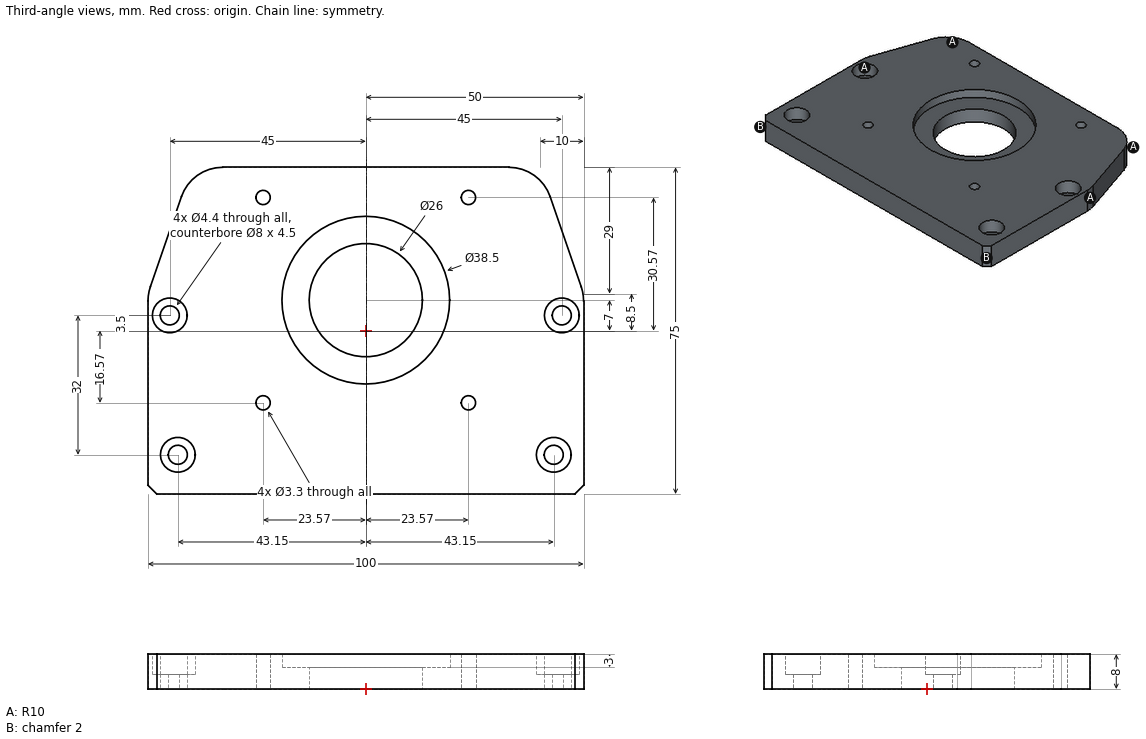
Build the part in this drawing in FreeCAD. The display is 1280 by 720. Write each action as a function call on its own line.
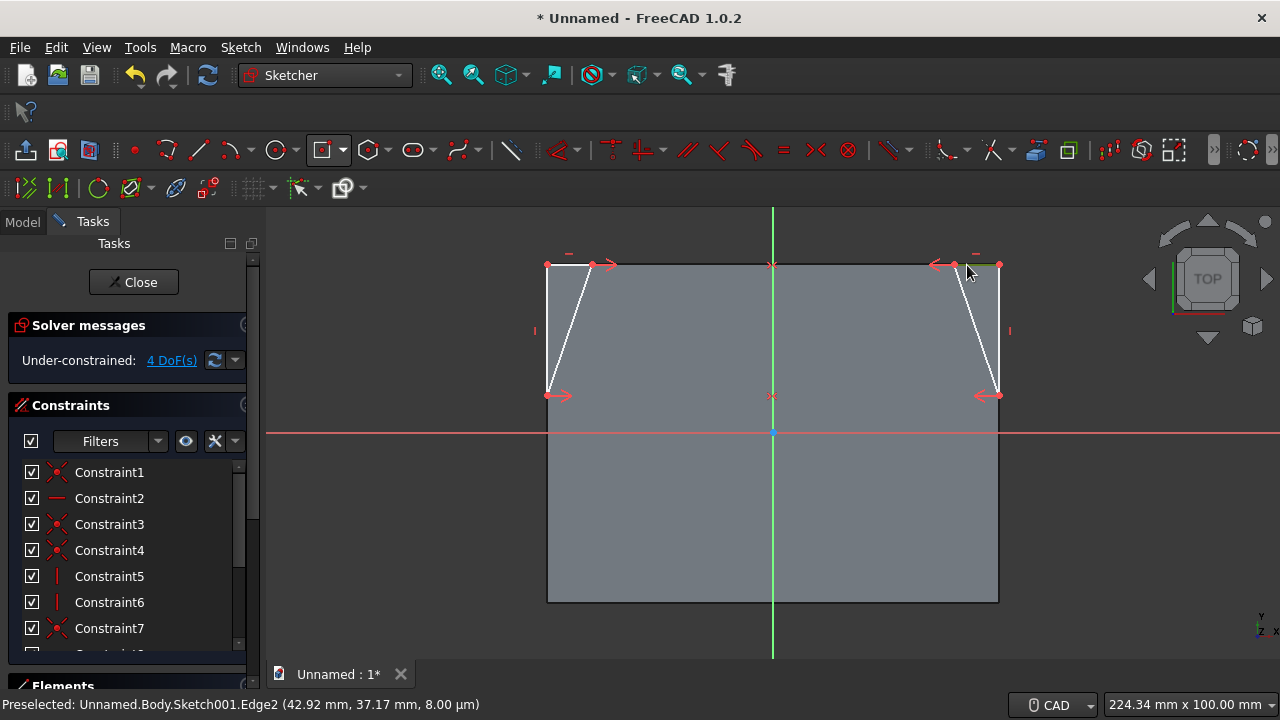
click(580, 150)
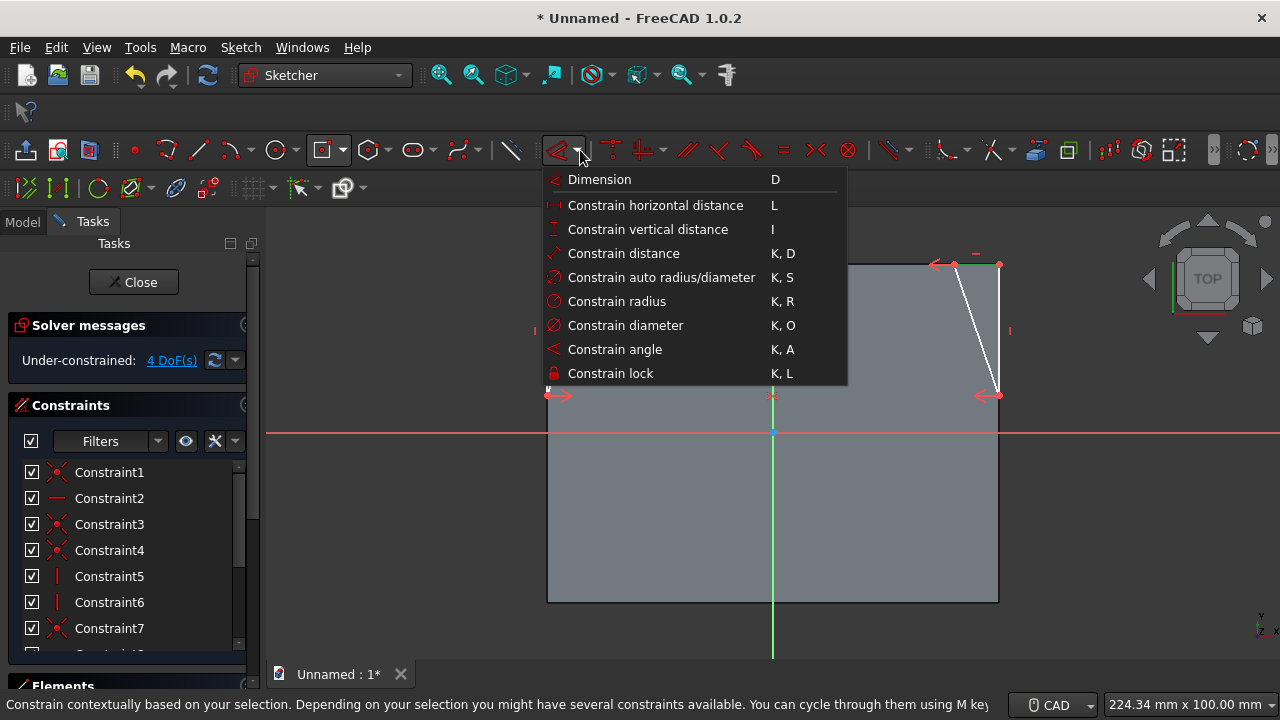
click(695, 205)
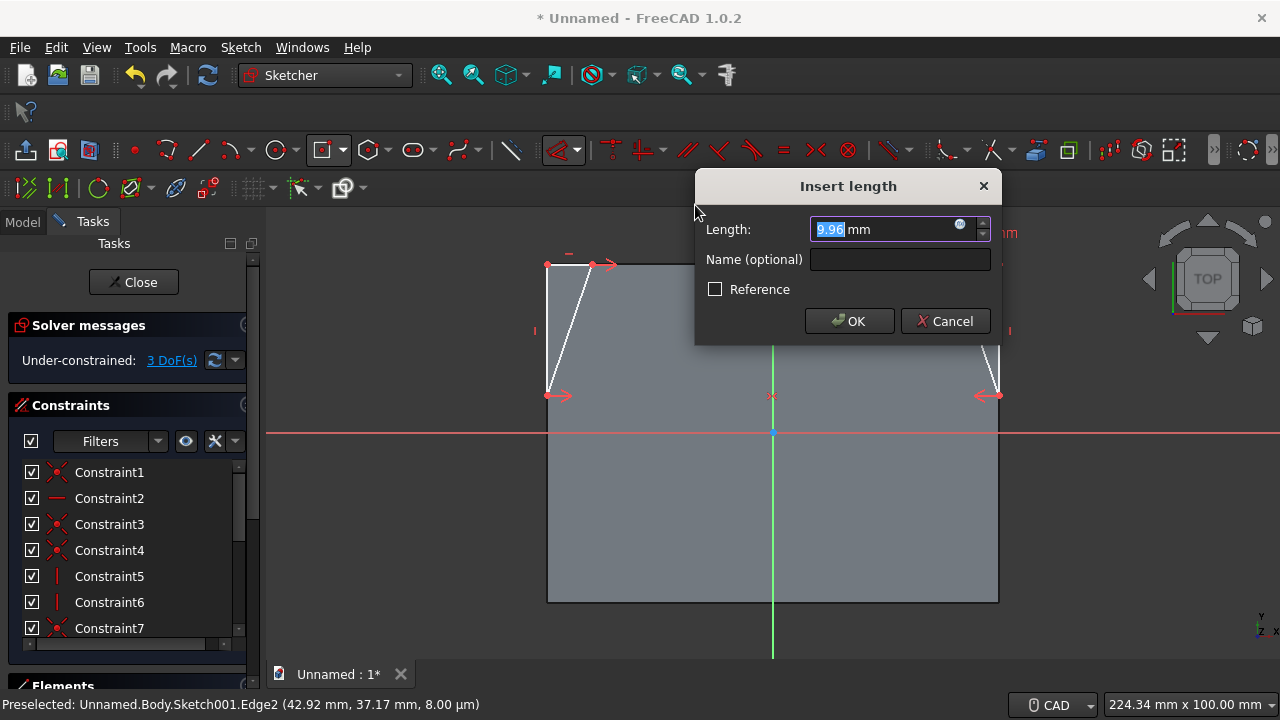
text(10)
key(Return)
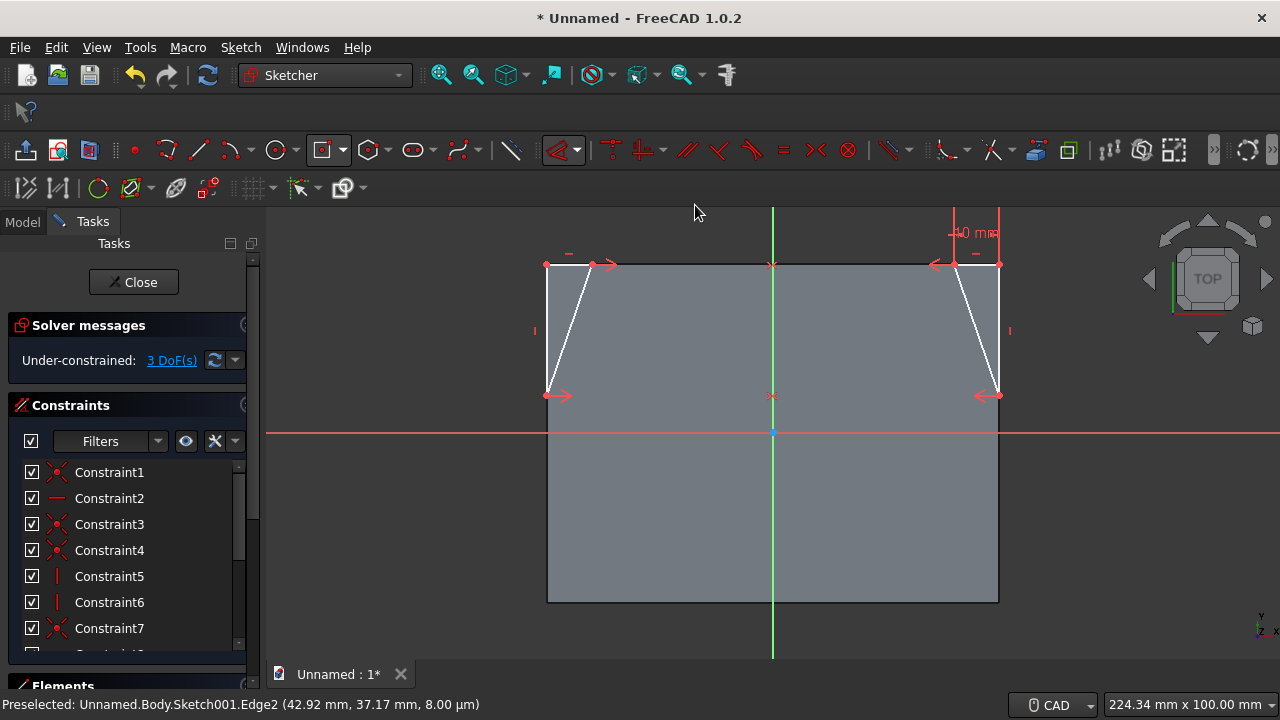
click(999, 304)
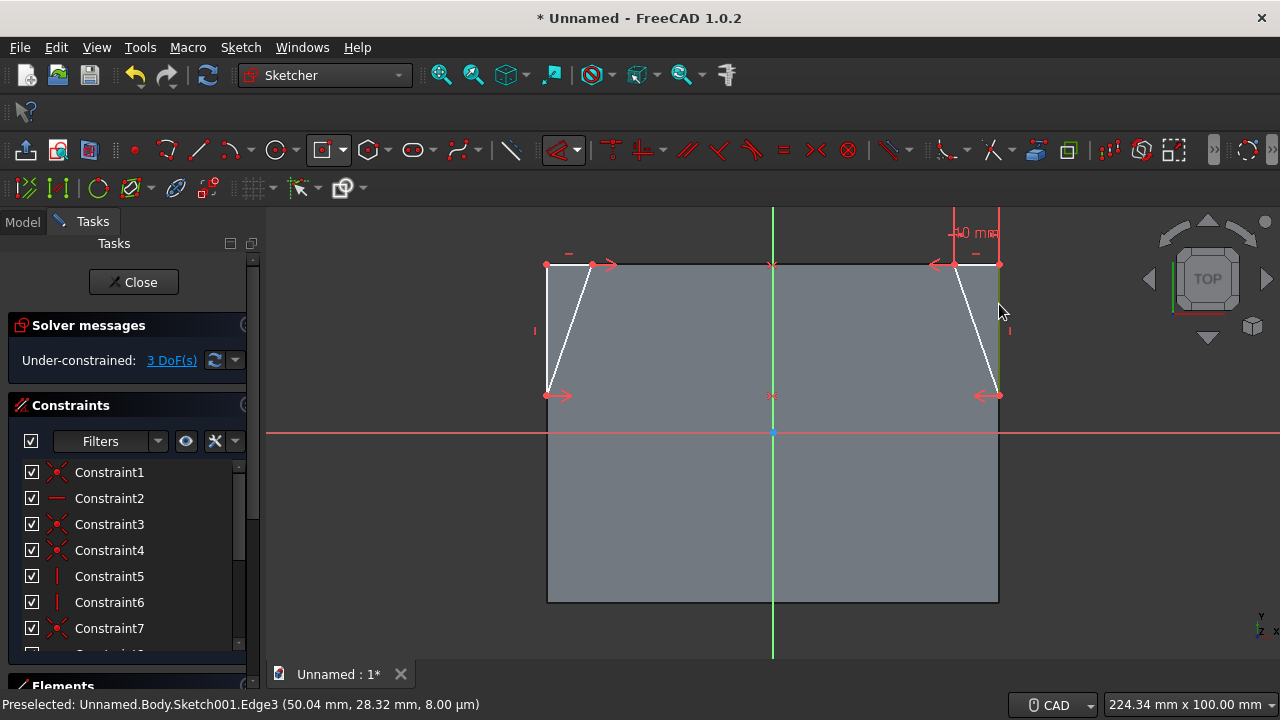
click(580, 150)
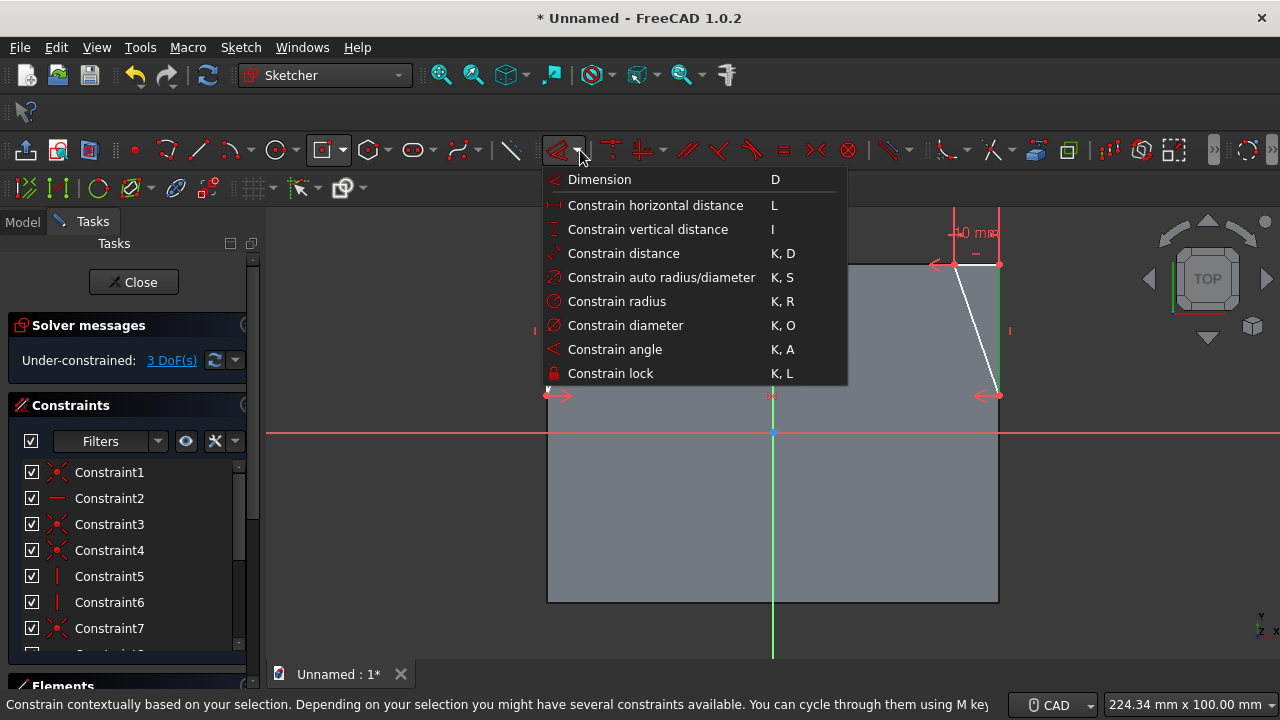
click(695, 229)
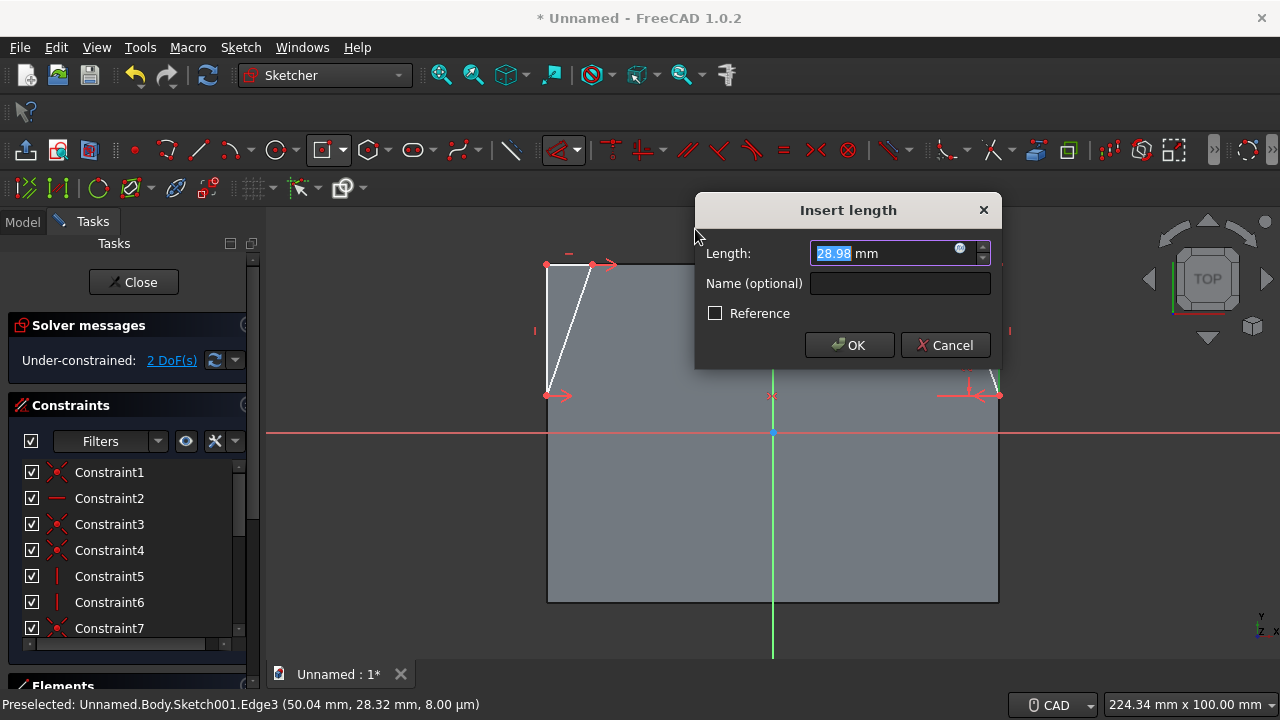
text(29)
key(Return)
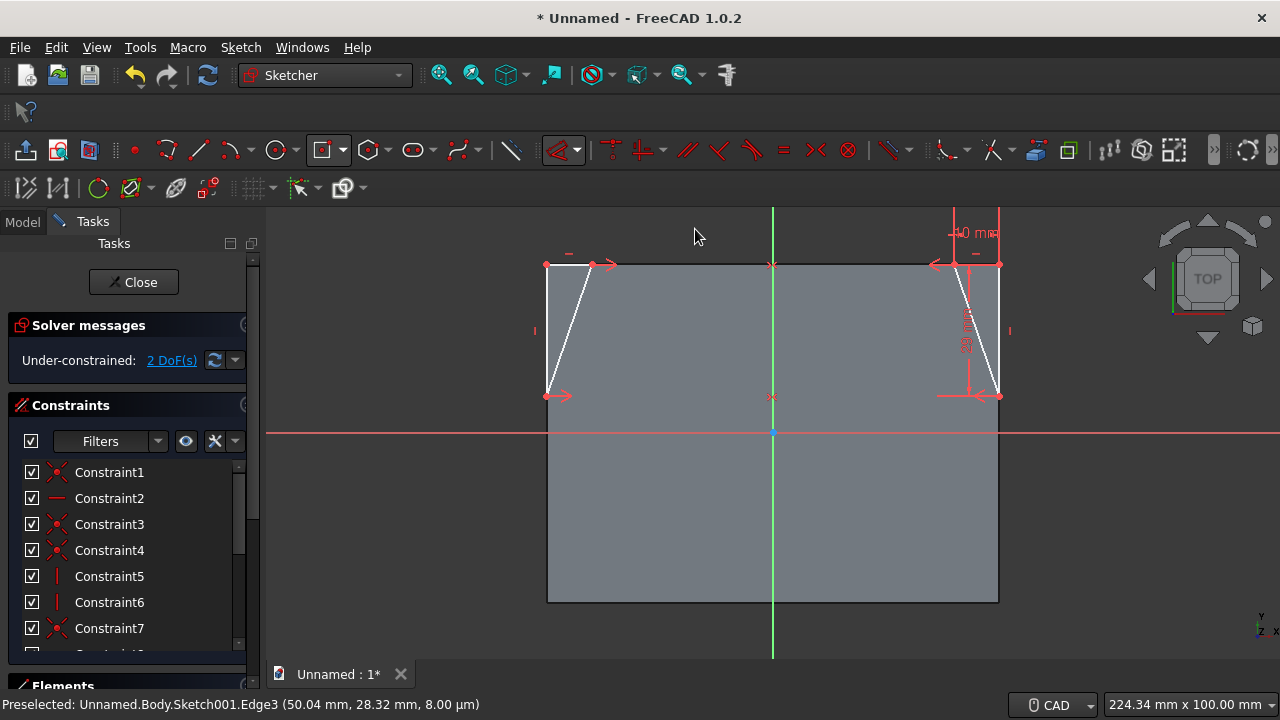
click(999, 396)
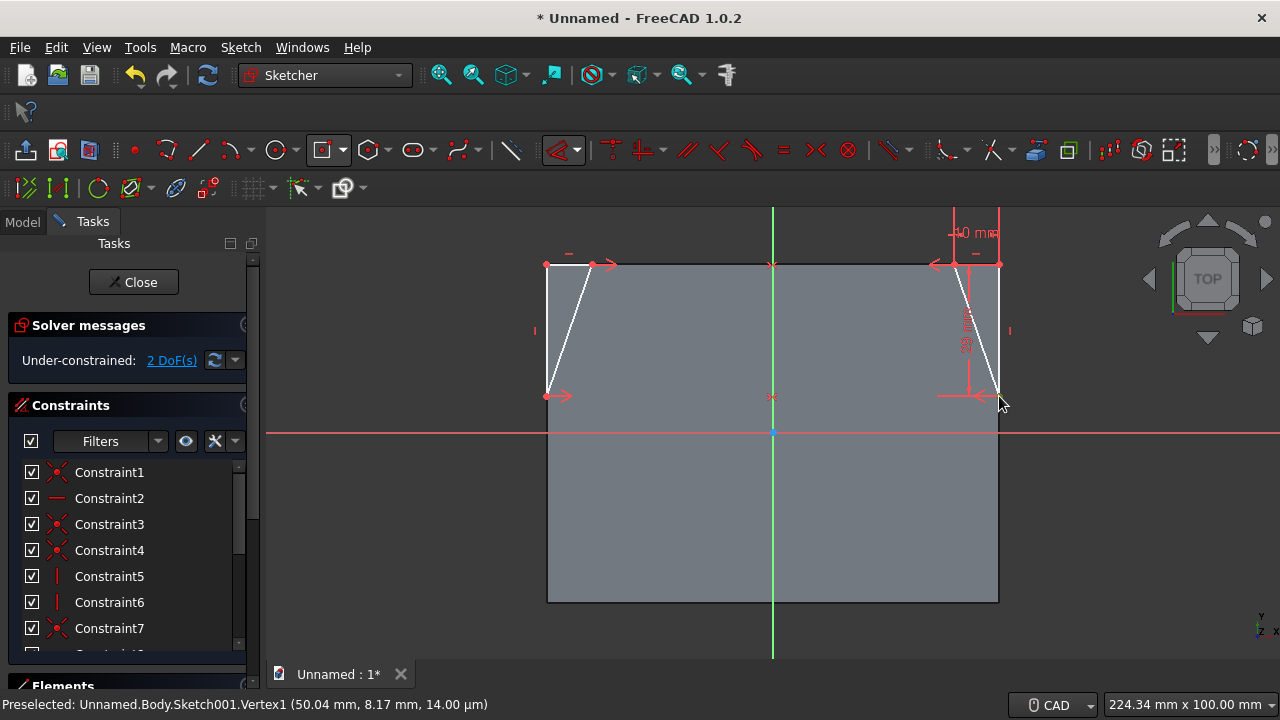
key(l)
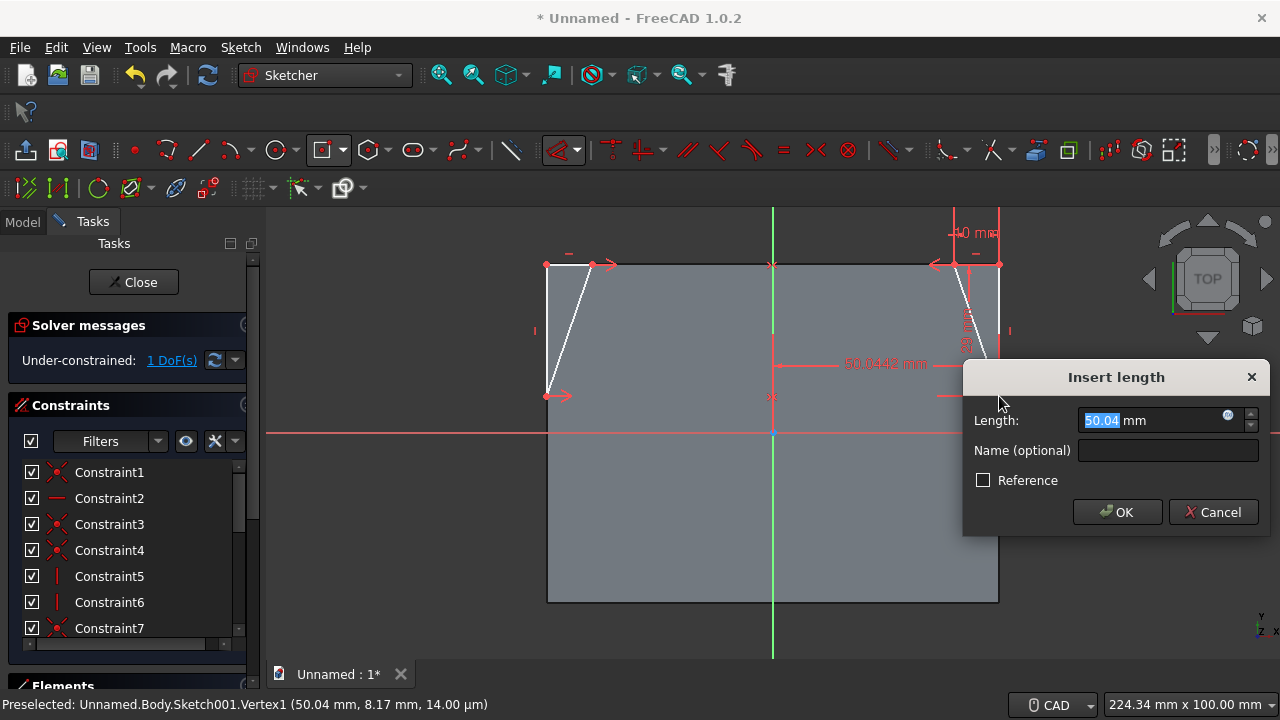
text(50)
key(Return)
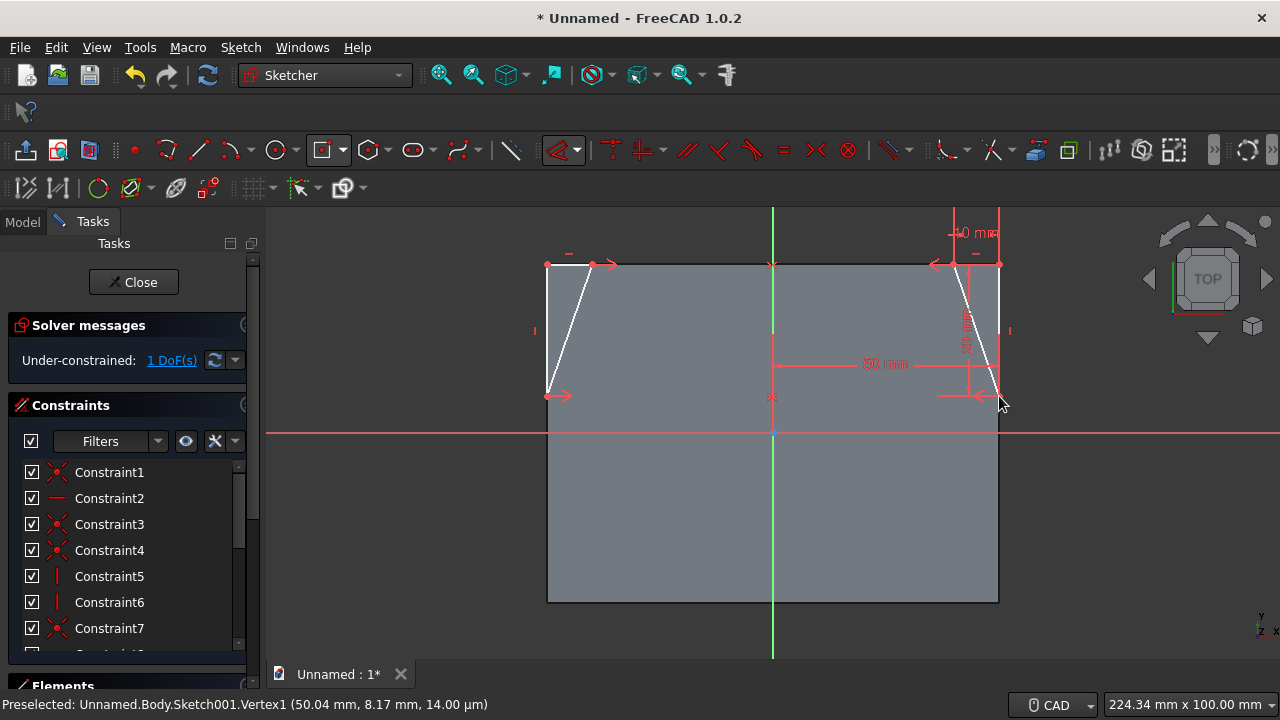
click(999, 396)